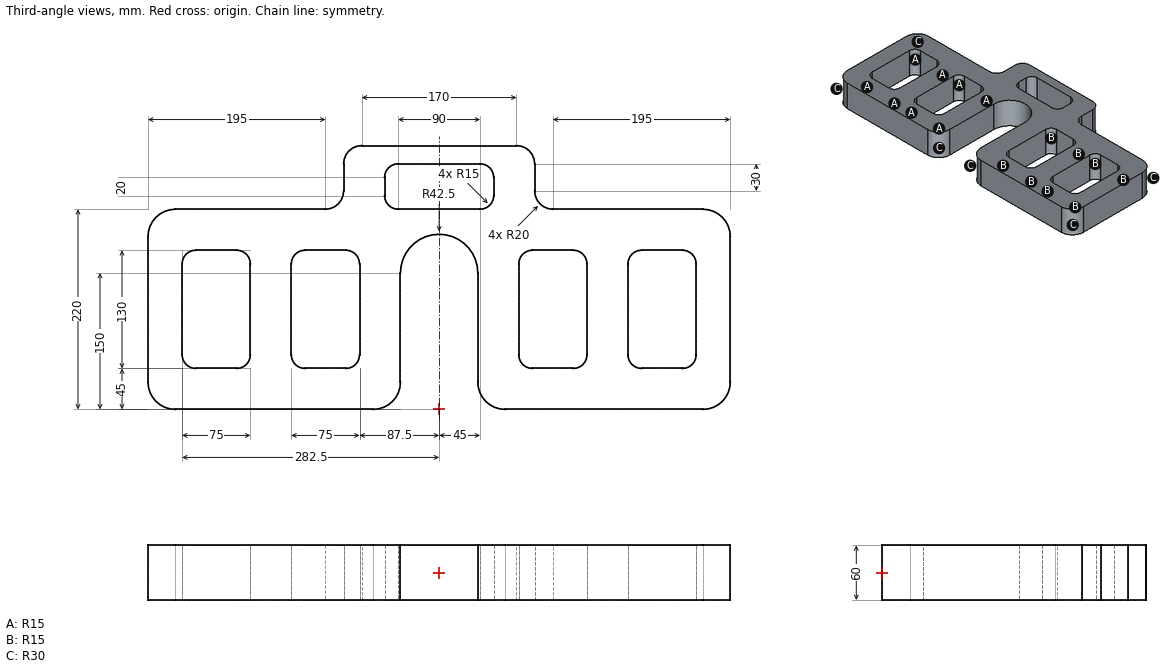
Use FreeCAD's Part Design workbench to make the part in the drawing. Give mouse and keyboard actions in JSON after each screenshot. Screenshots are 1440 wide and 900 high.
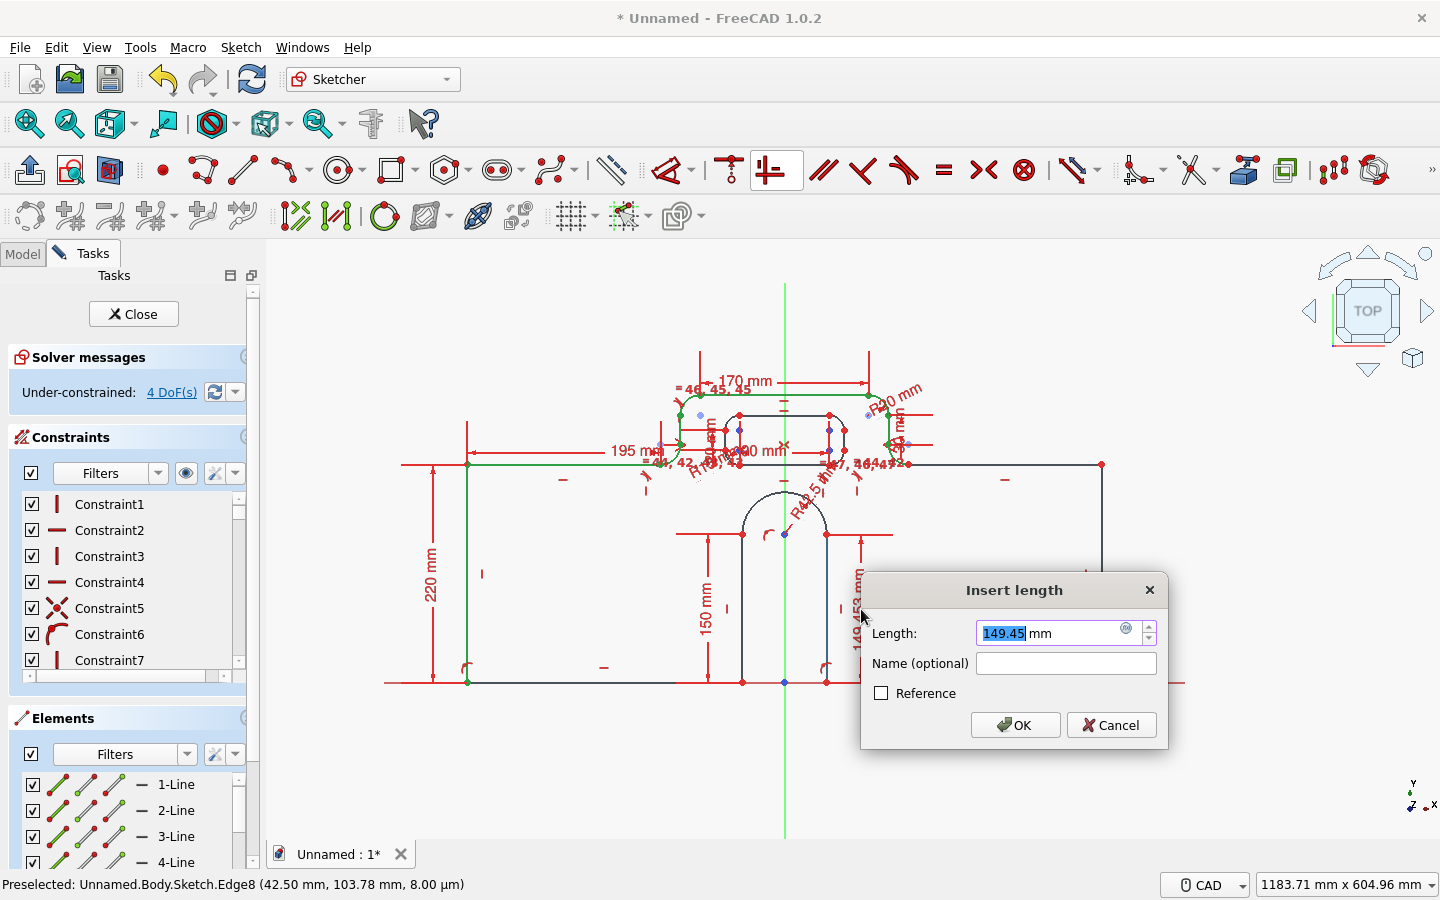
{"action": "type", "text": "150"}
{"action": "key", "text": "Return"}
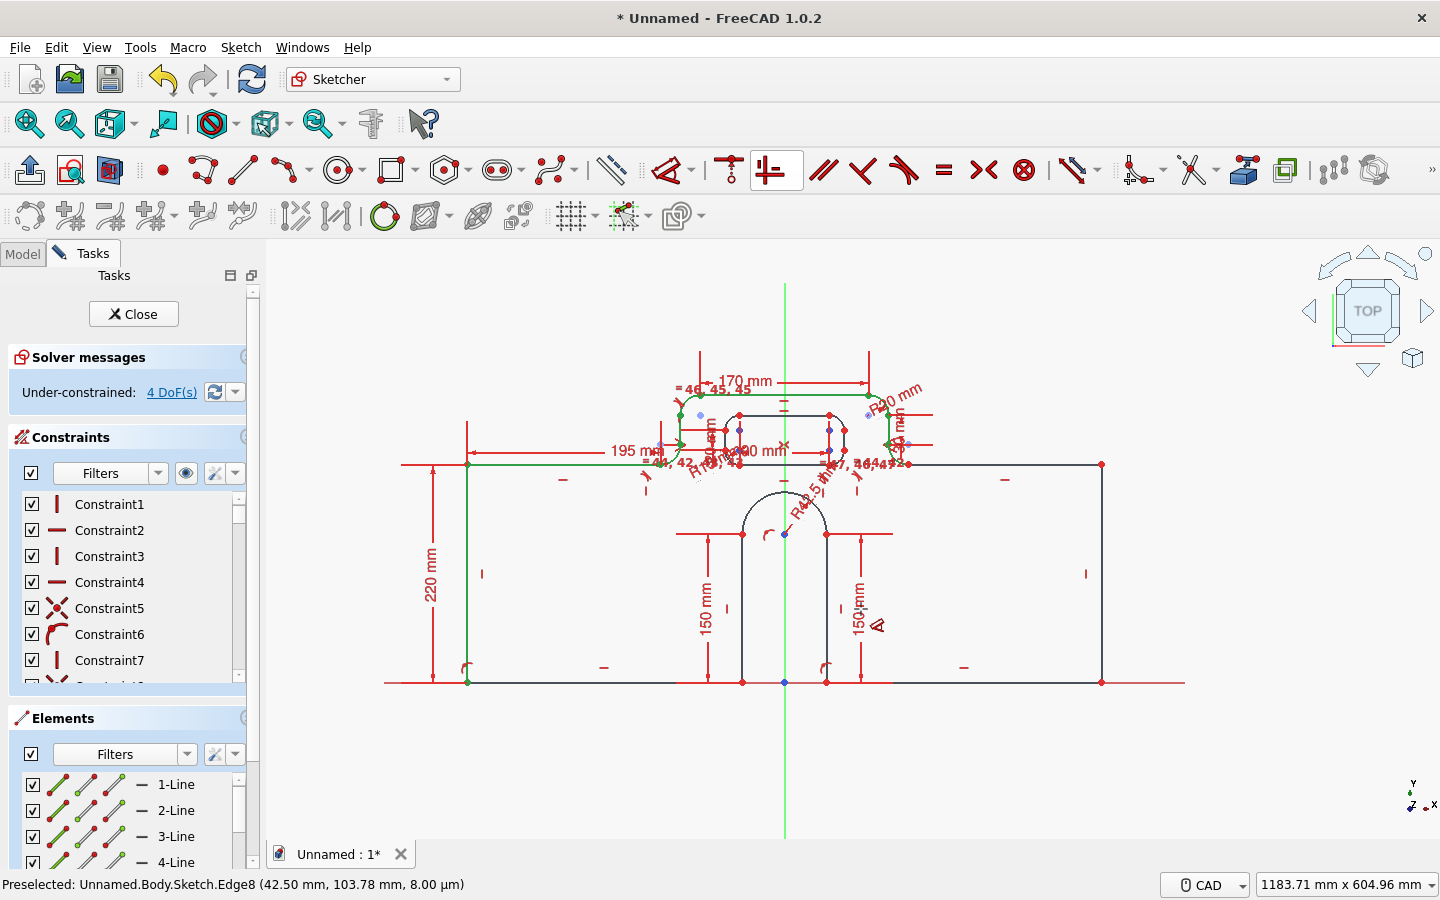
{"action": "left_click", "coordinate": [1044, 465]}
{"action": "left_click", "coordinate": [1005, 431]}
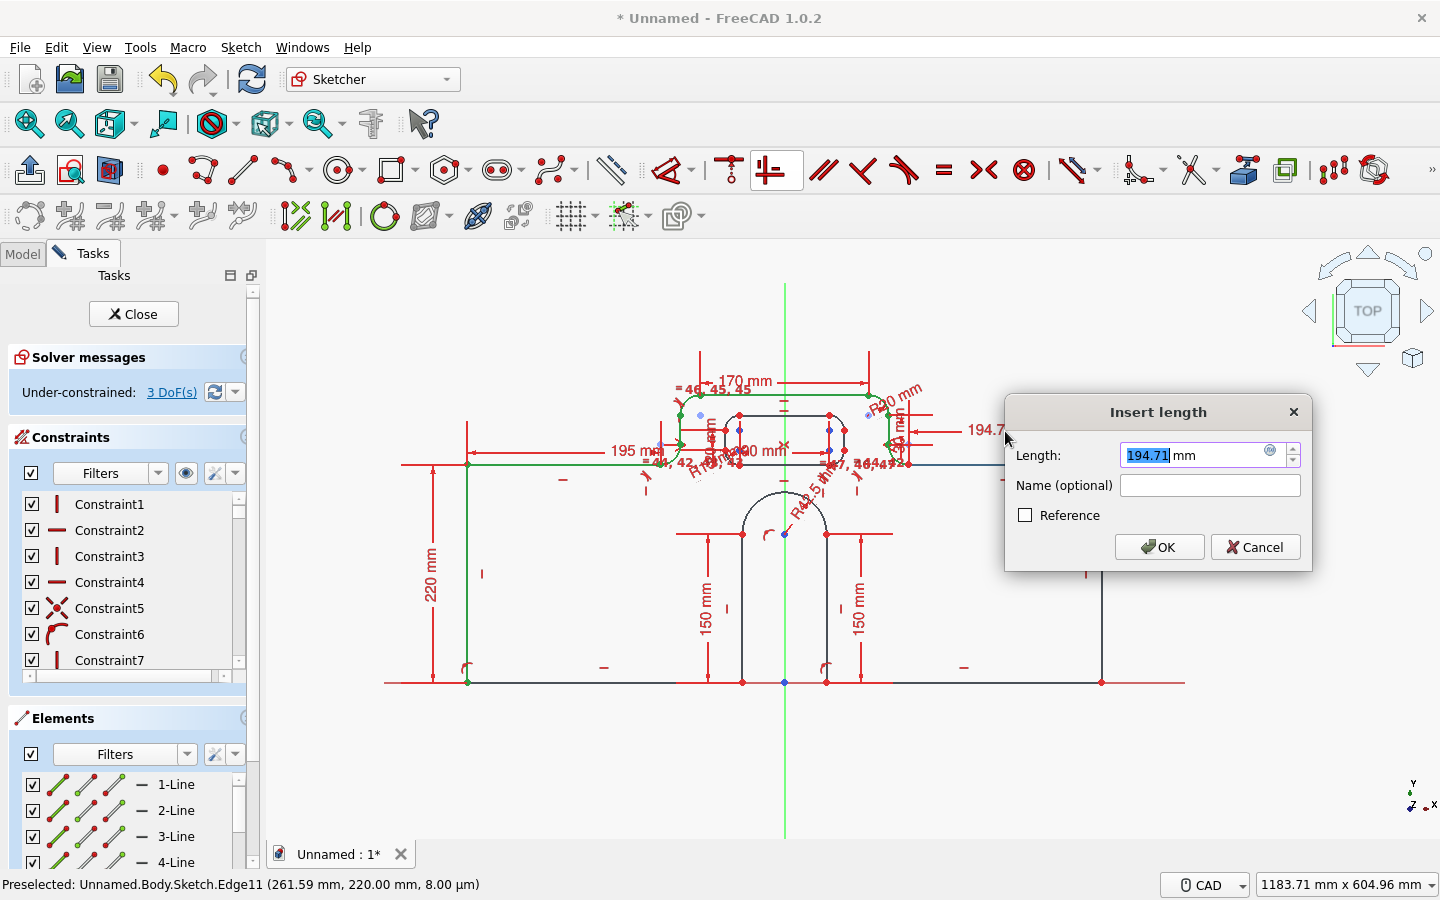
{"action": "type", "text": "195"}
{"action": "key", "text": "Return"}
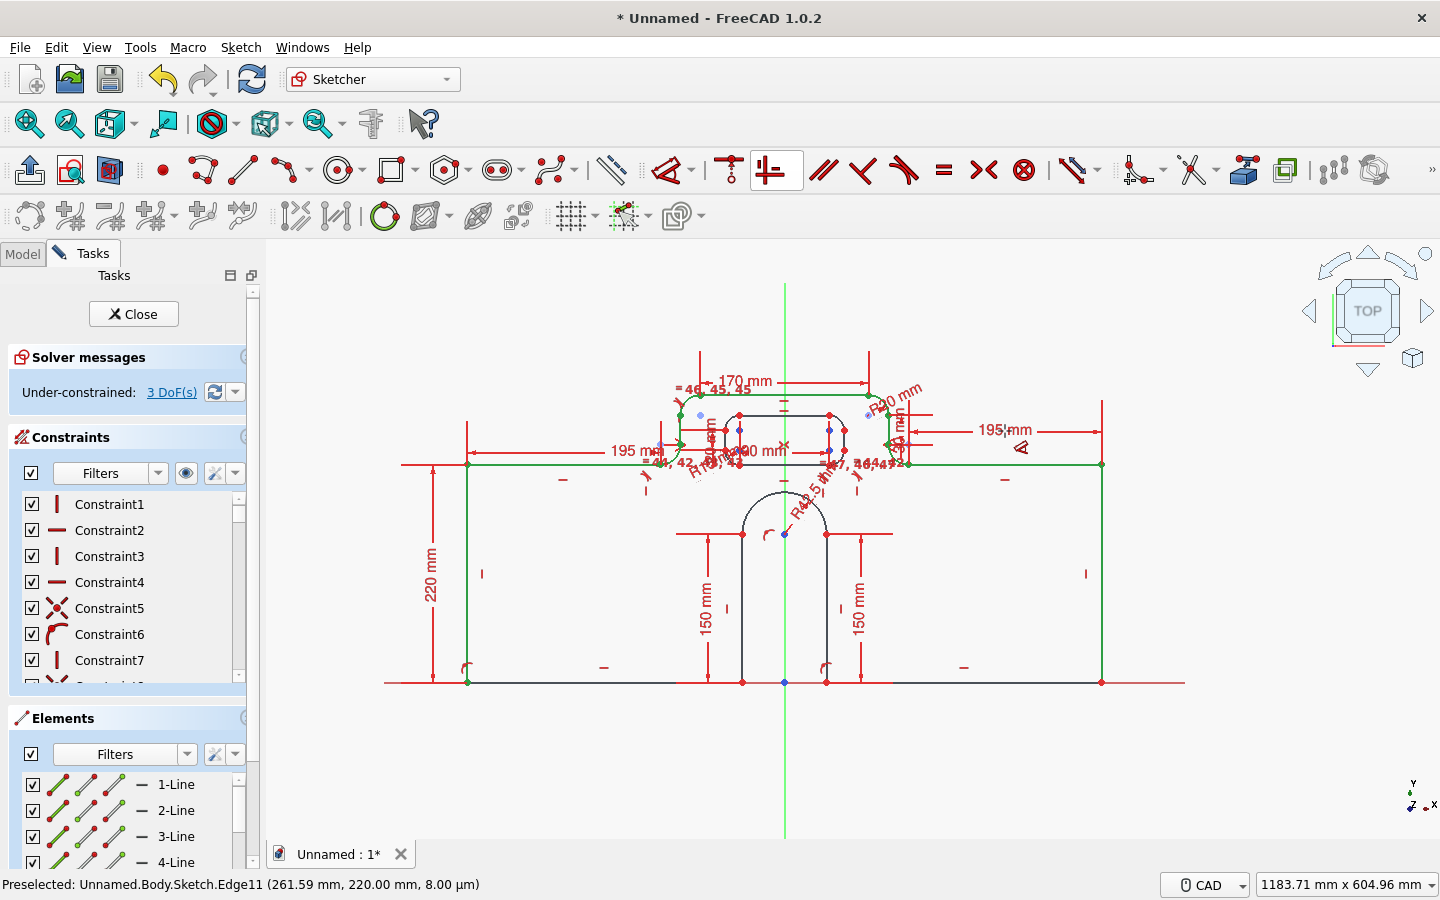
{"action": "left_click", "coordinate": [829, 465]}
{"action": "left_click", "coordinate": [807, 717]}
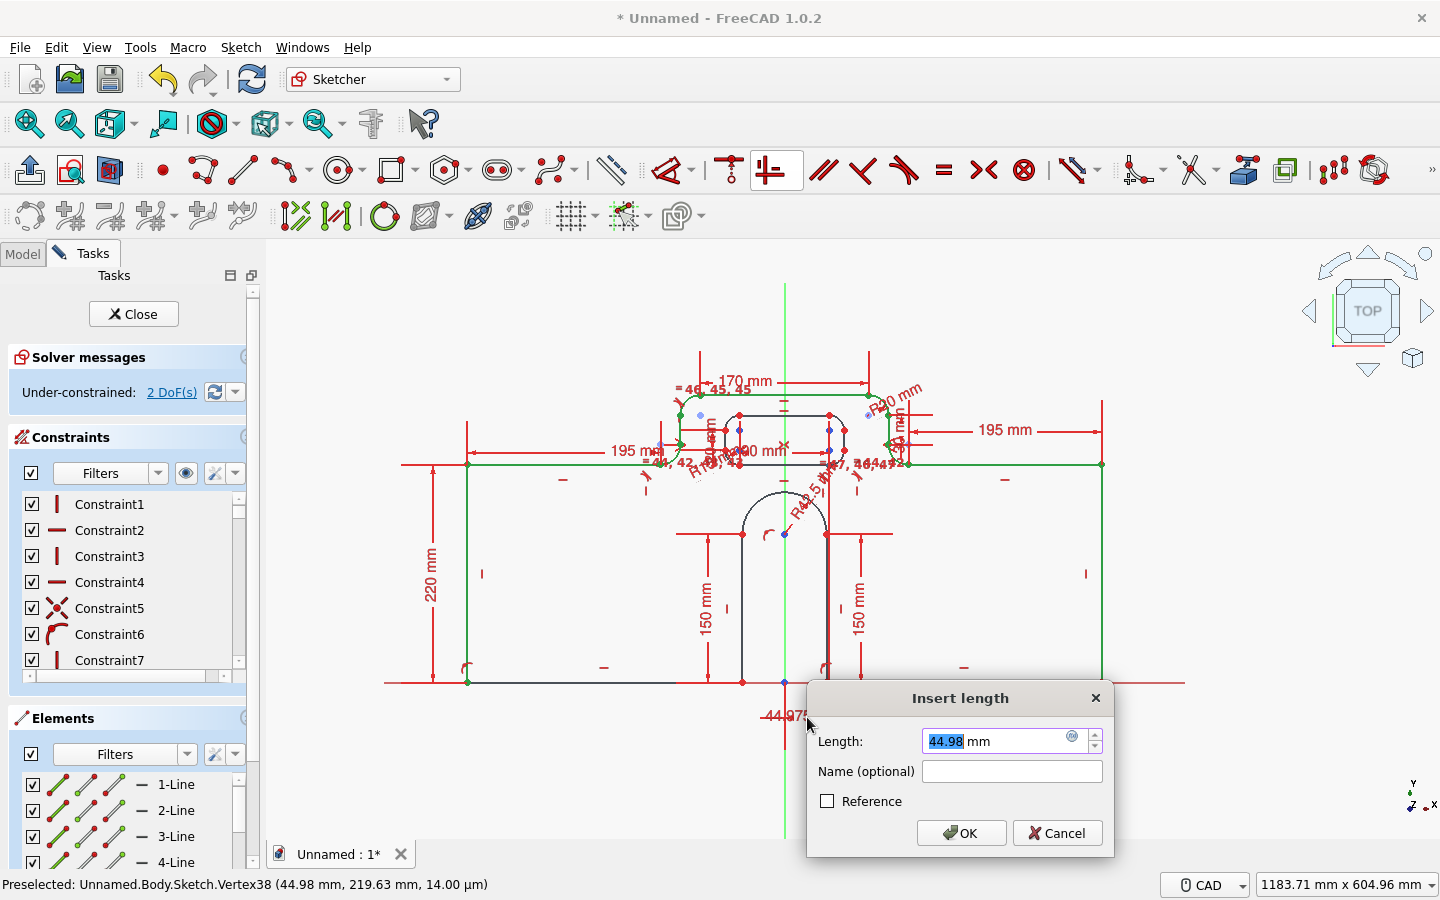
{"action": "type", "text": "45"}
{"action": "key", "text": "Return"}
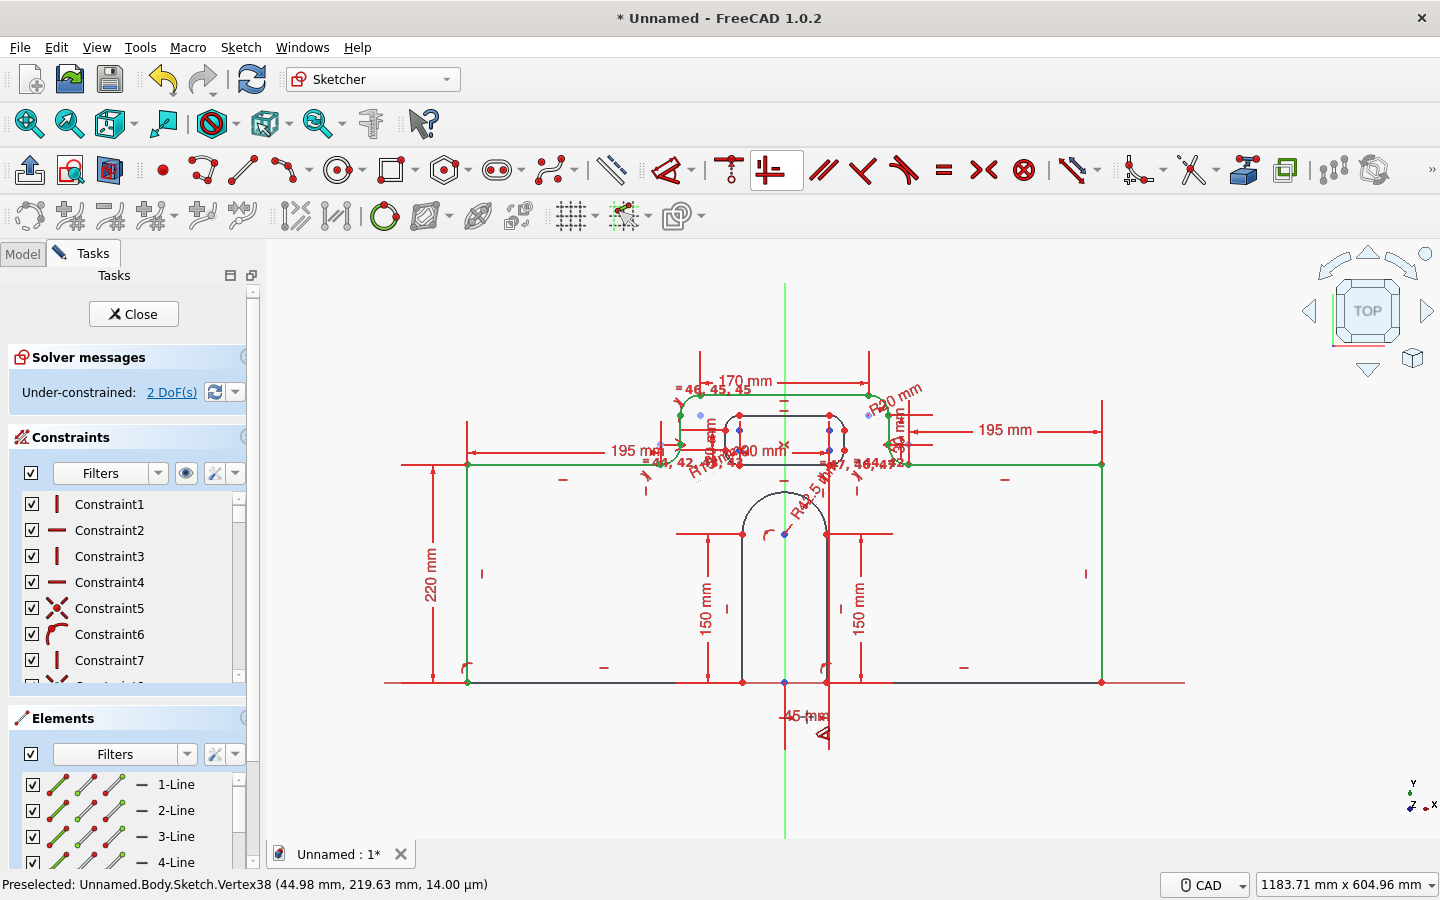
{"action": "left_click", "coordinate": [829, 465]}
{"action": "left_click", "coordinate": [863, 574]}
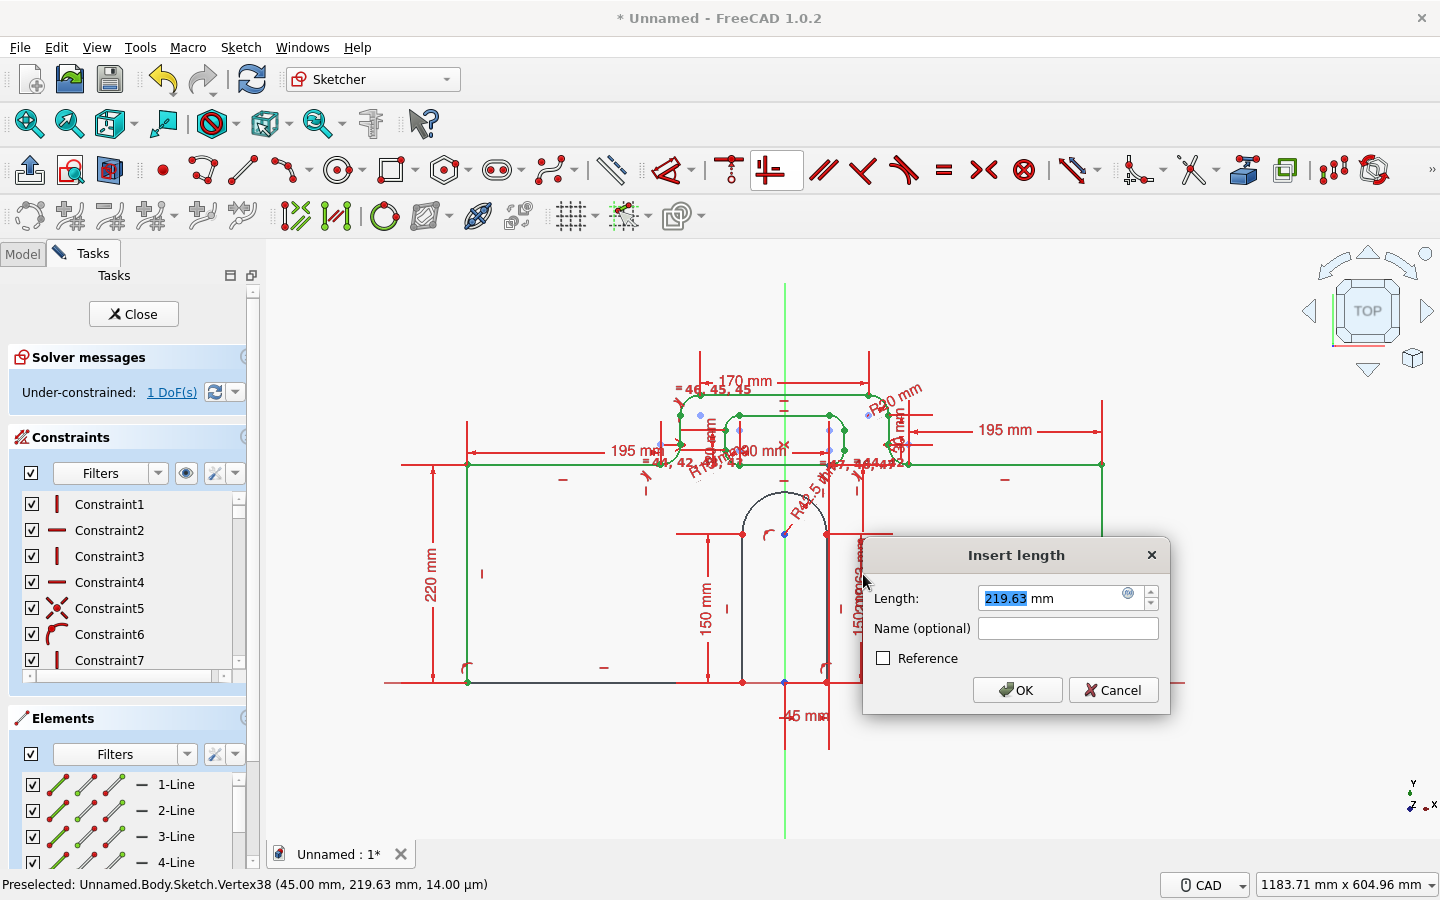
{"action": "type", "text": "220"}
{"action": "key", "text": "Return"}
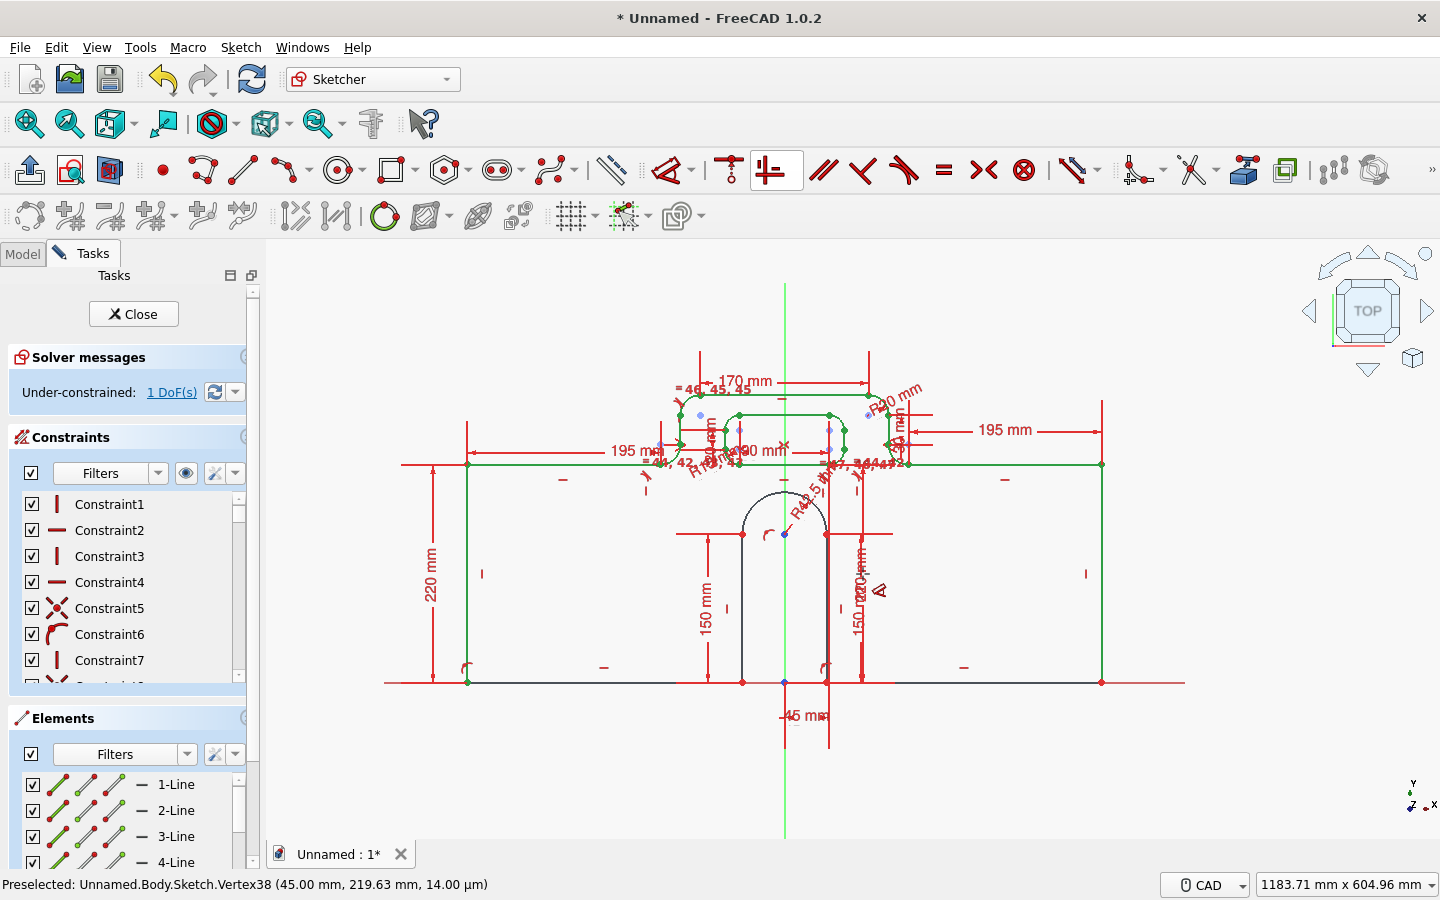
{"action": "left_click", "coordinate": [785, 534]}
{"action": "left_click", "coordinate": [843, 643]}